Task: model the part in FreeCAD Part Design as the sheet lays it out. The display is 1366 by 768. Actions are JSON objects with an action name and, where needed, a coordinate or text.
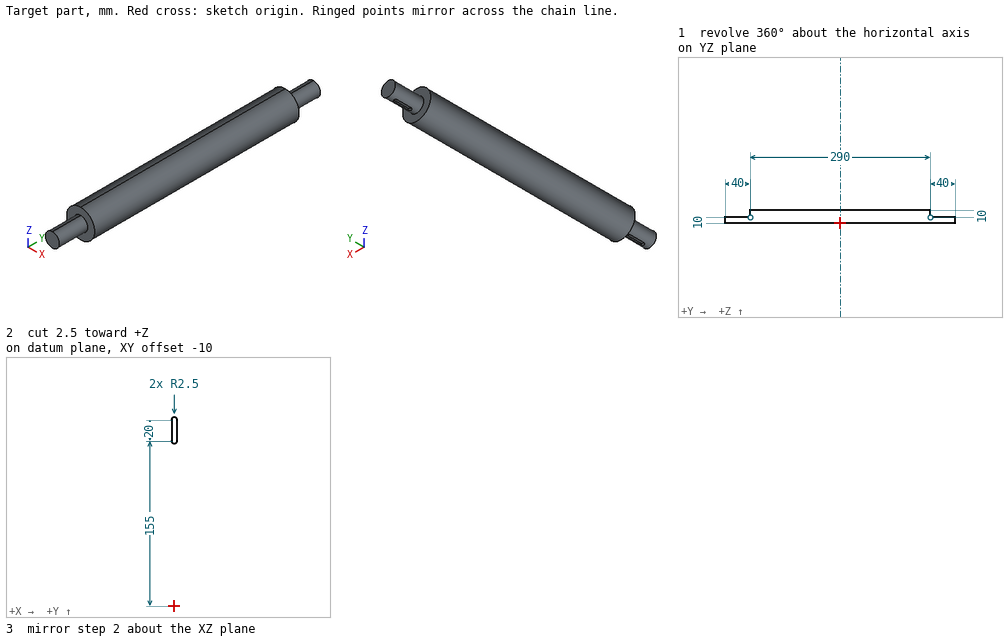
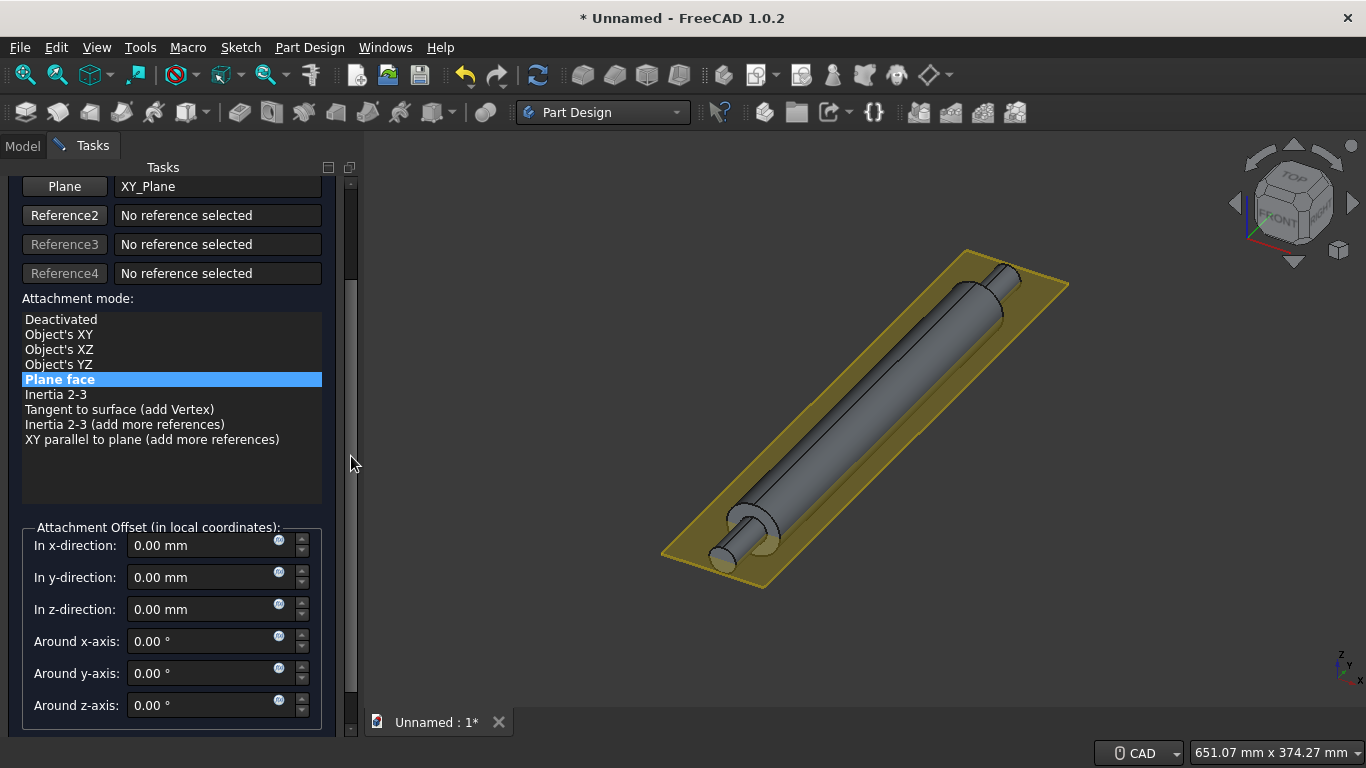
{"action": "triple_click", "coordinate": [210, 609]}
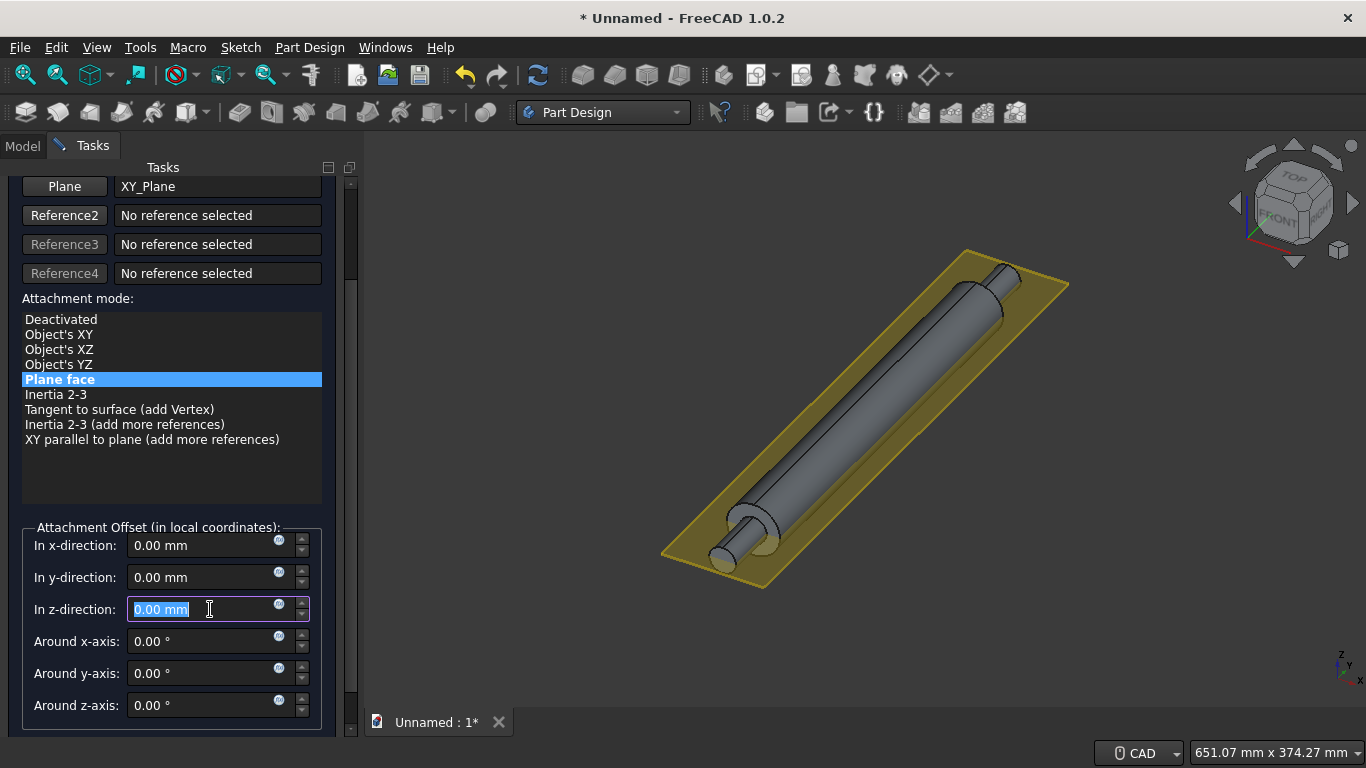
{"action": "type", "text": "-10"}
{"action": "key", "text": "Tab"}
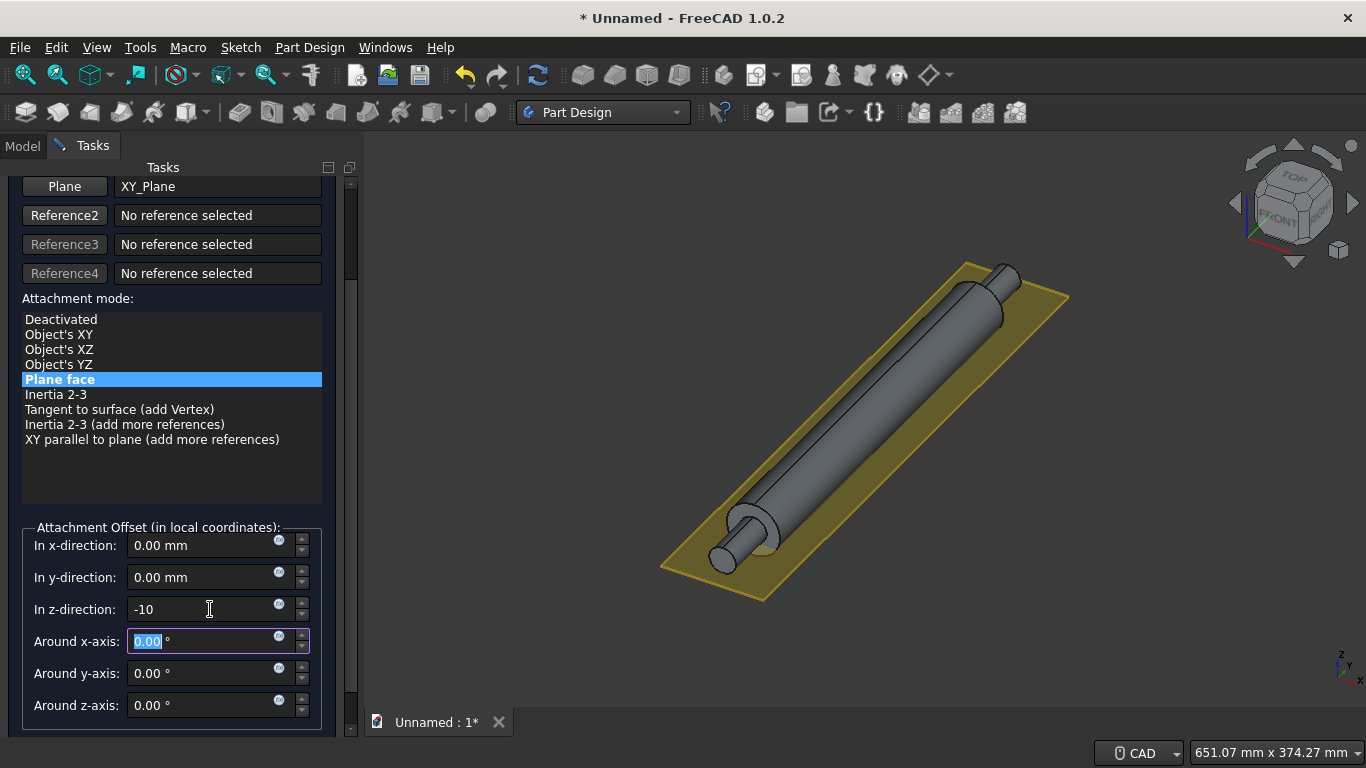
{"action": "scroll", "coordinate": [351, 456], "scroll_direction": "up", "scroll_amount": 3}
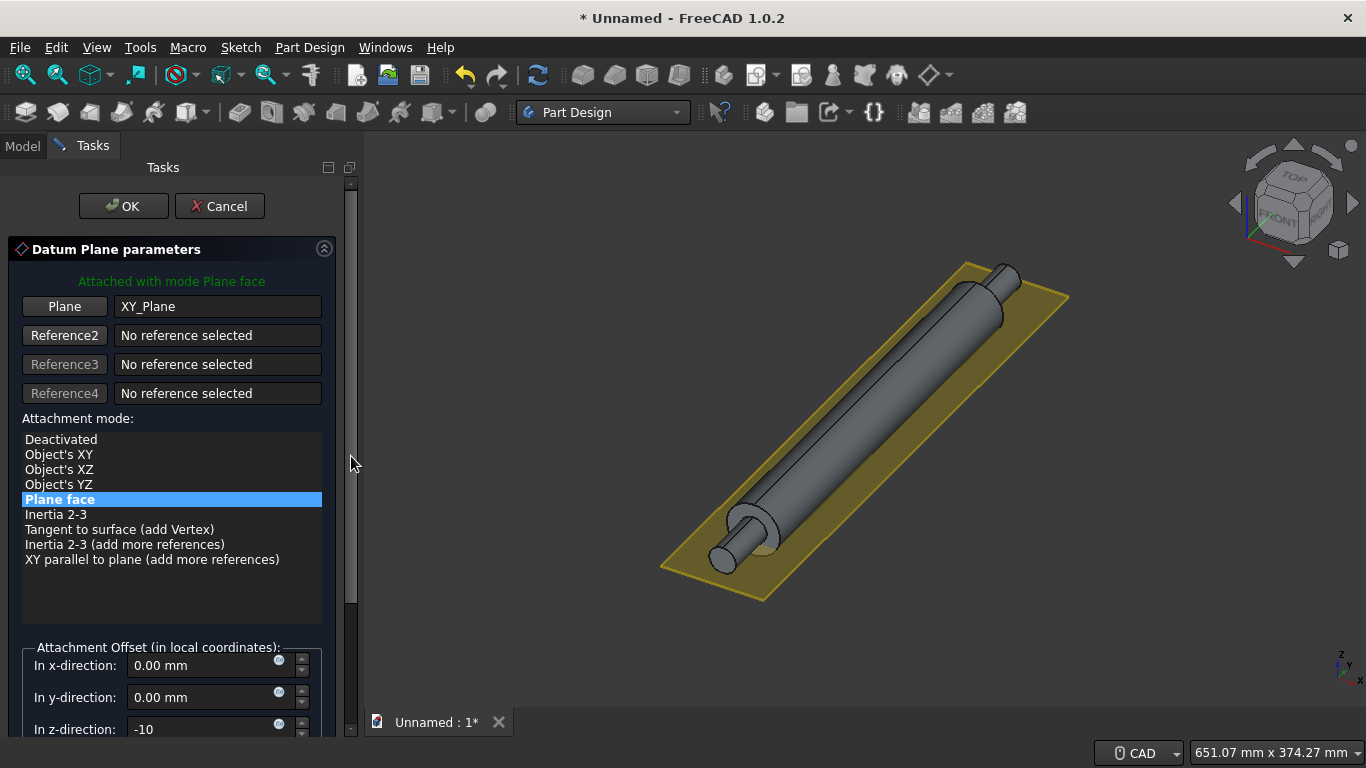
{"action": "left_click", "coordinate": [124, 206]}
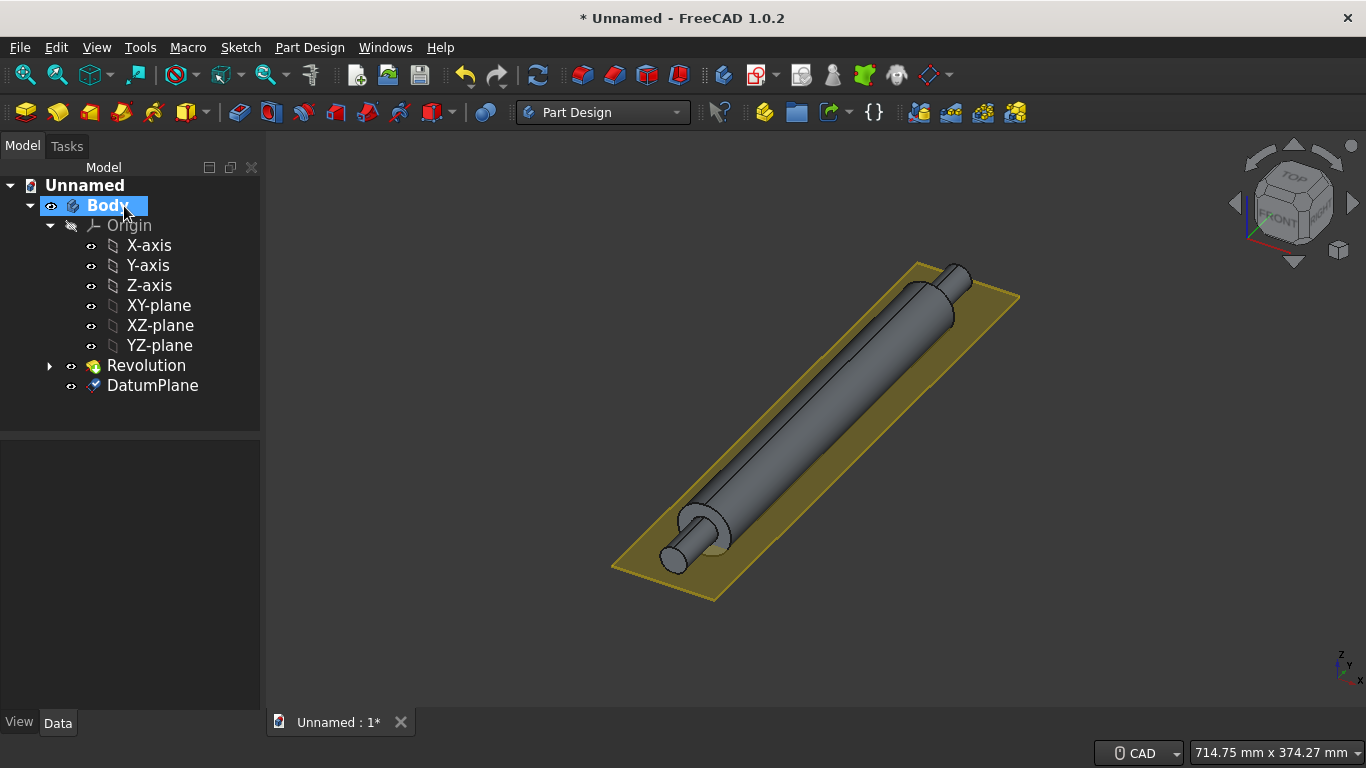
{"action": "left_click", "coordinate": [116, 386]}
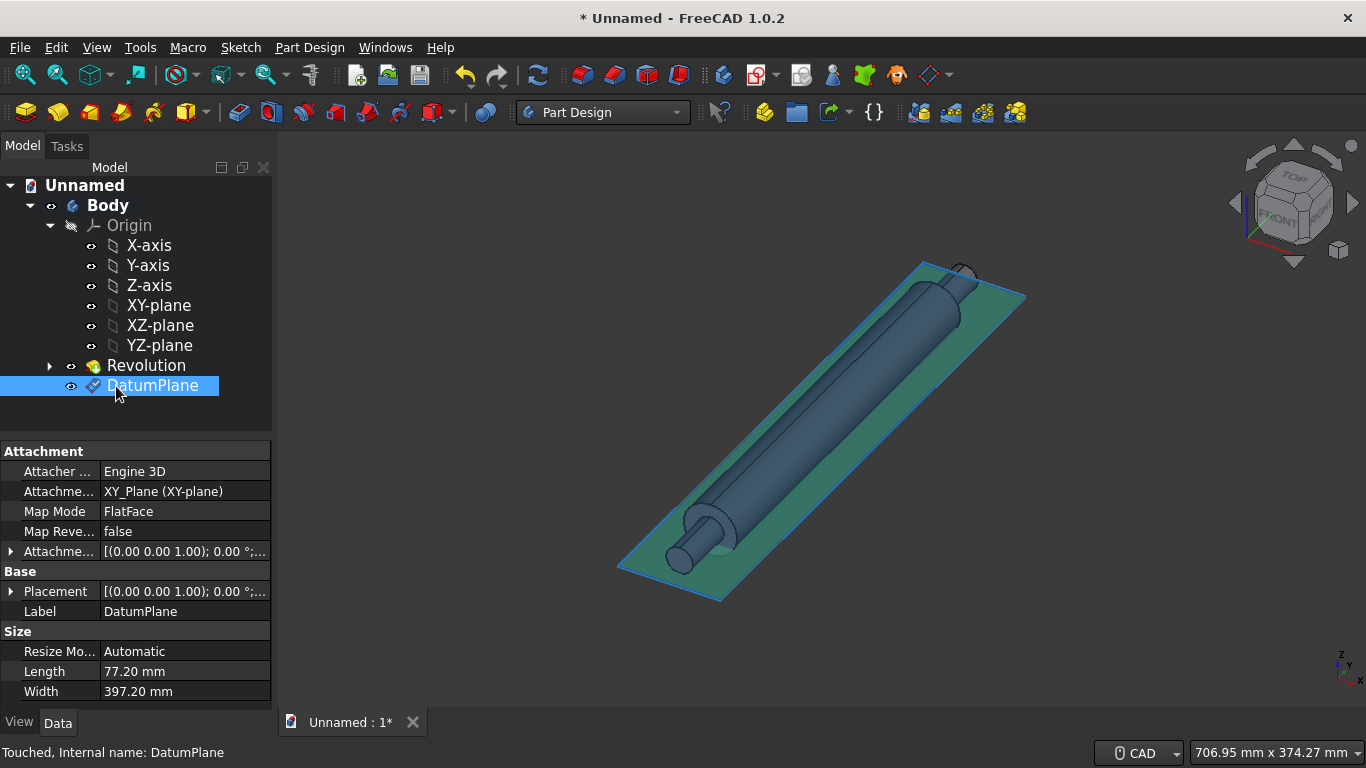
{"action": "left_click", "coordinate": [756, 76]}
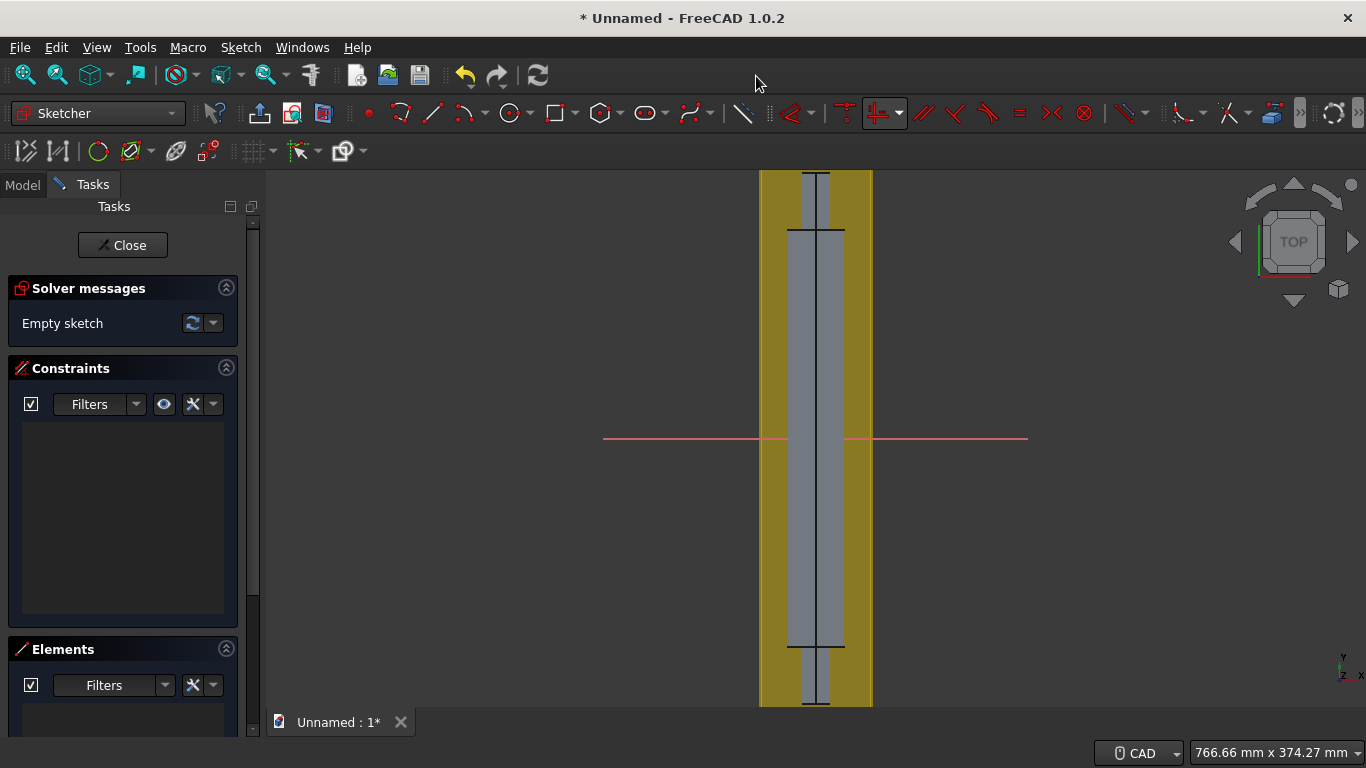
{"action": "left_click", "coordinate": [324, 114]}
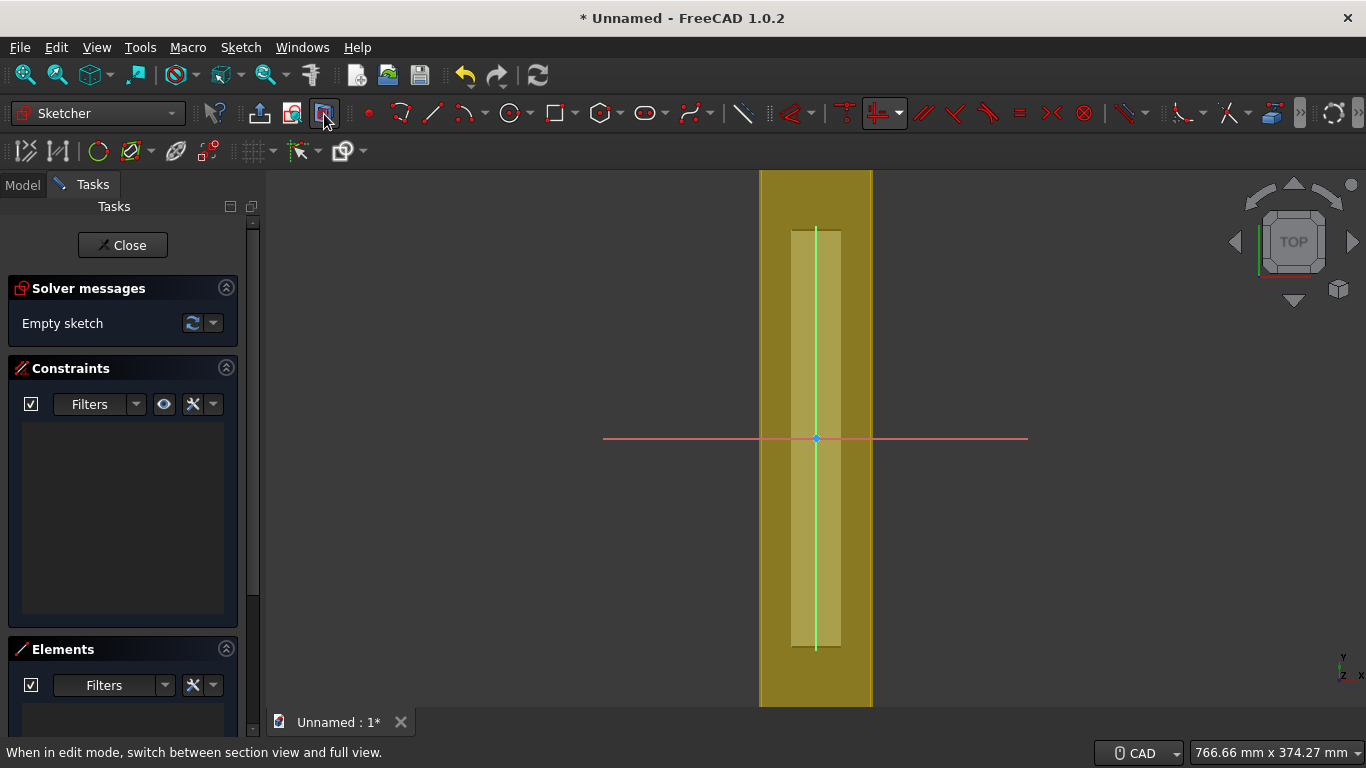
{"action": "scroll", "coordinate": [748, 438], "scroll_direction": "down", "scroll_amount": 5}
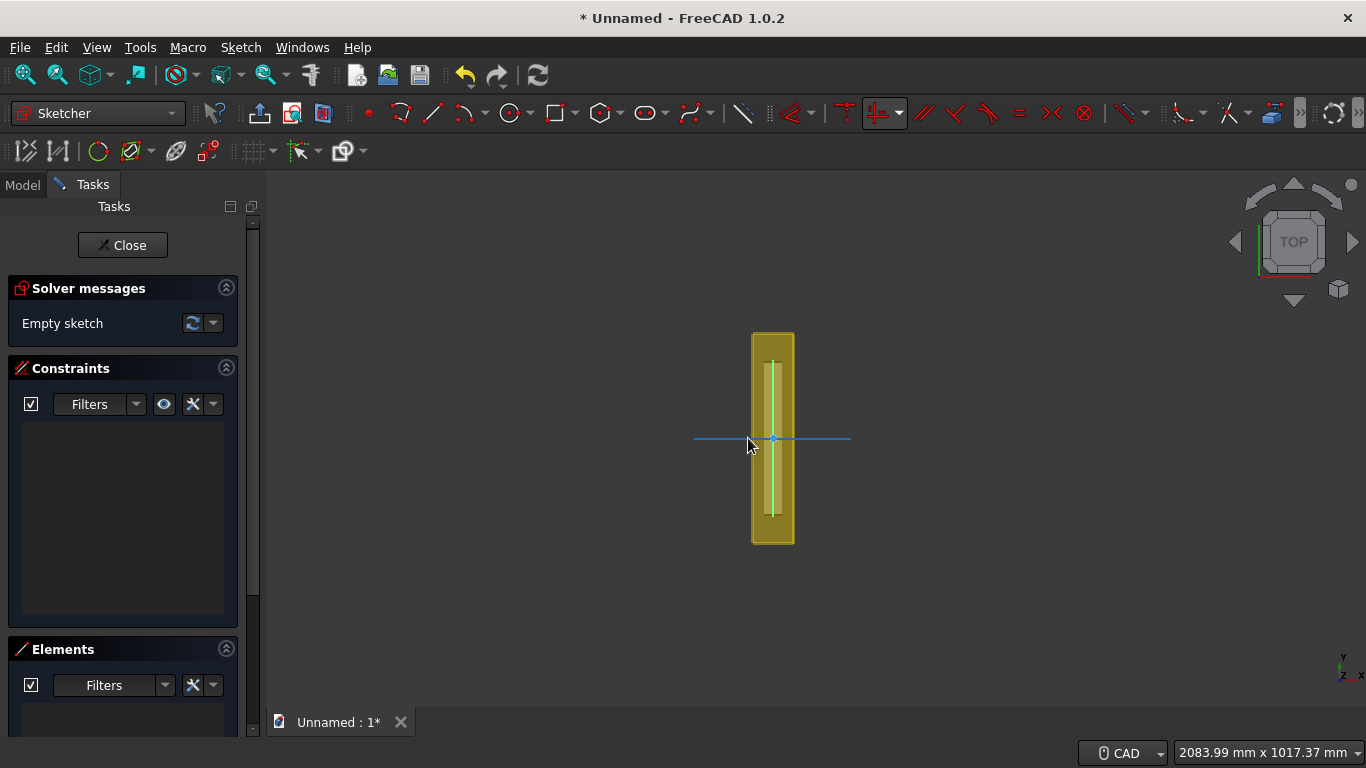
{"action": "scroll", "coordinate": [775, 347], "scroll_direction": "up", "scroll_amount": 15}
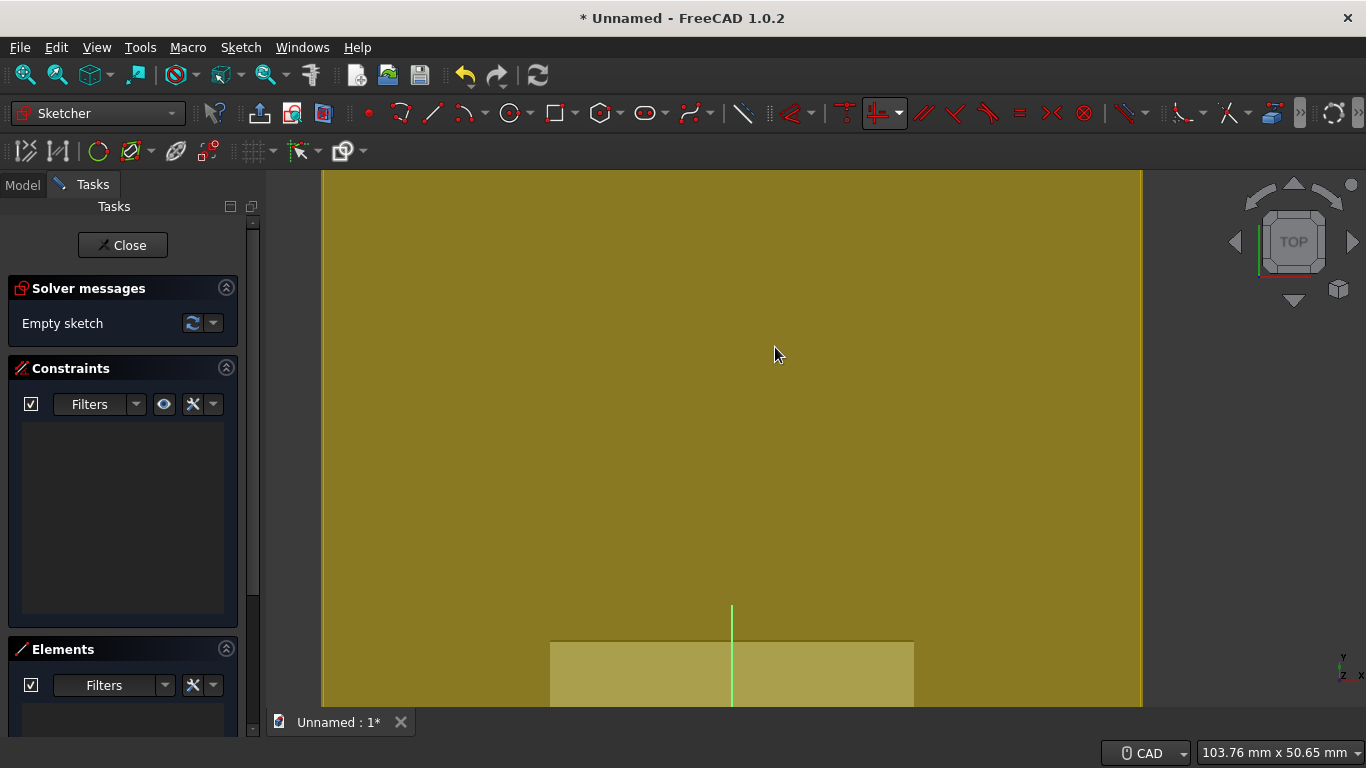
{"action": "key", "text": "g s"}